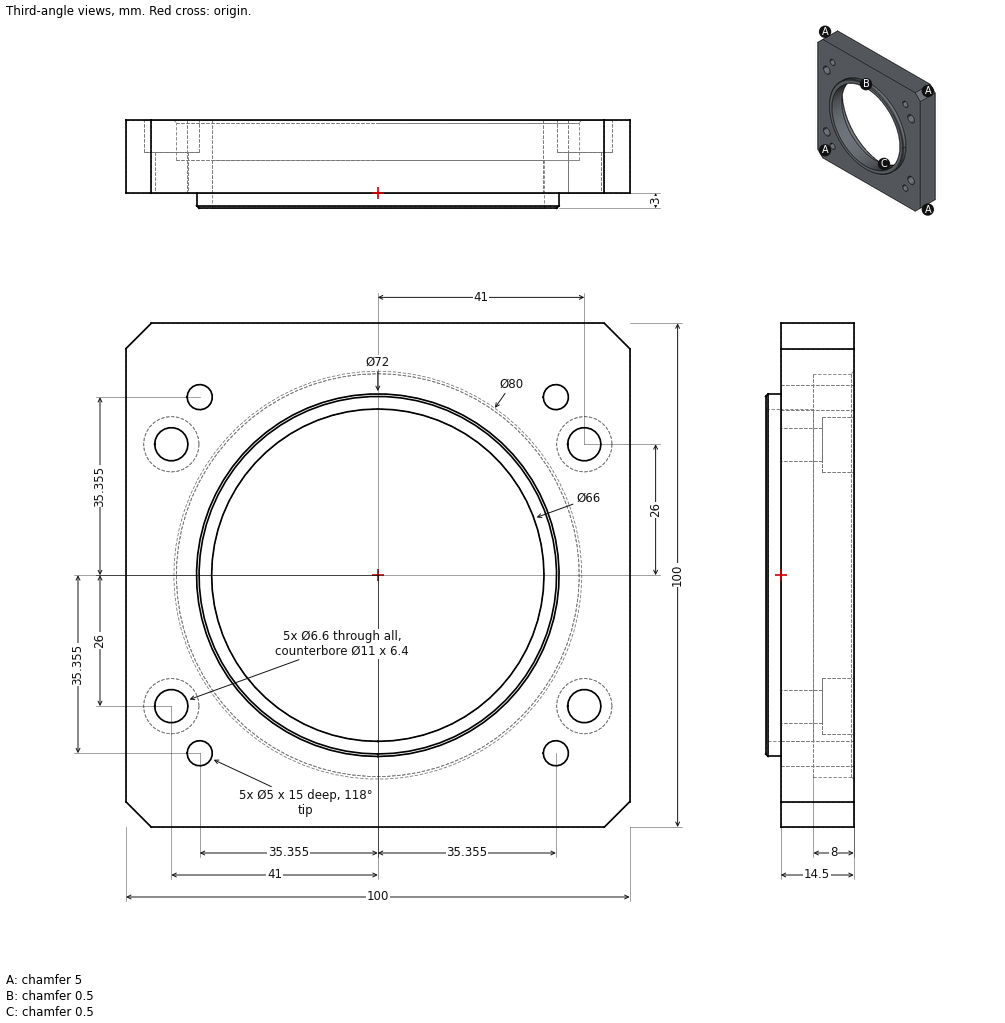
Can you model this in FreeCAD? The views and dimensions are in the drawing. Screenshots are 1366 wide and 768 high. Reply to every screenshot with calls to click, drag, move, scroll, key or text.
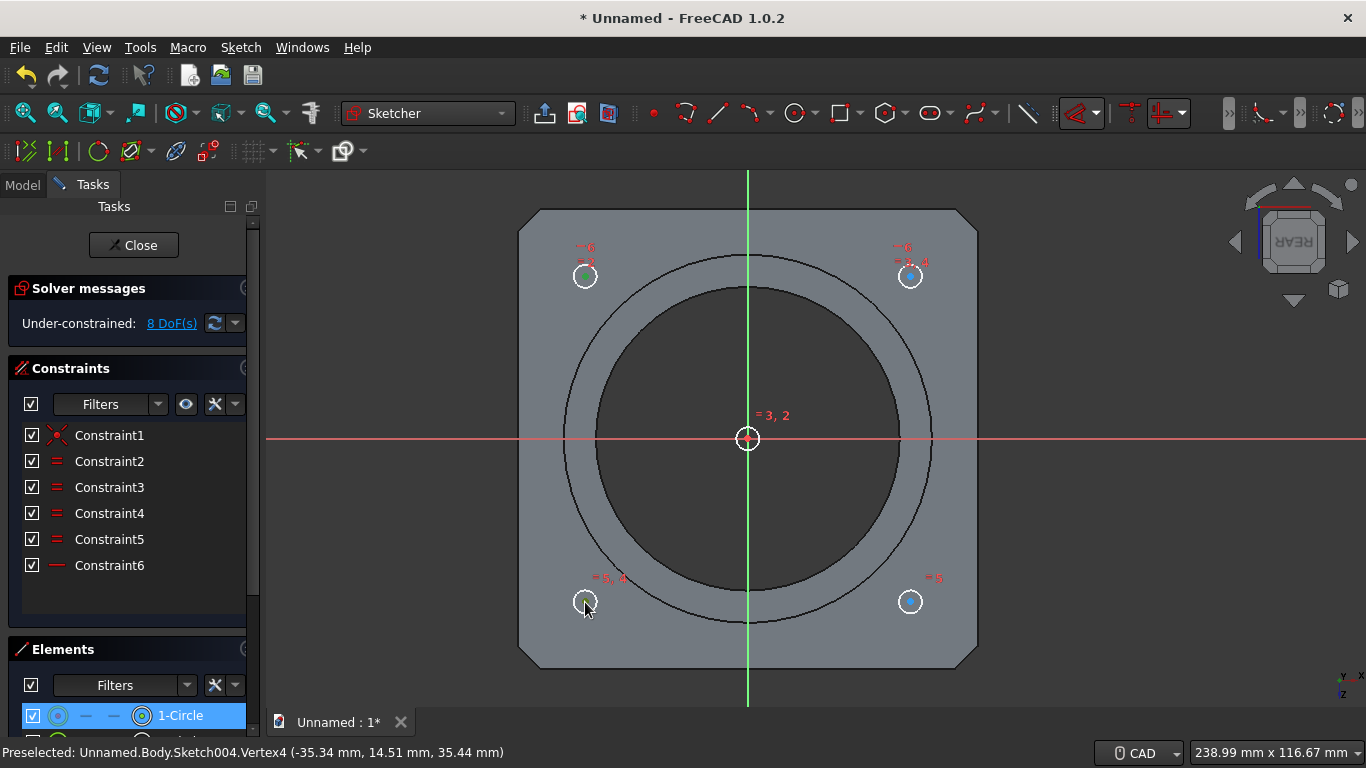
click(1184, 114)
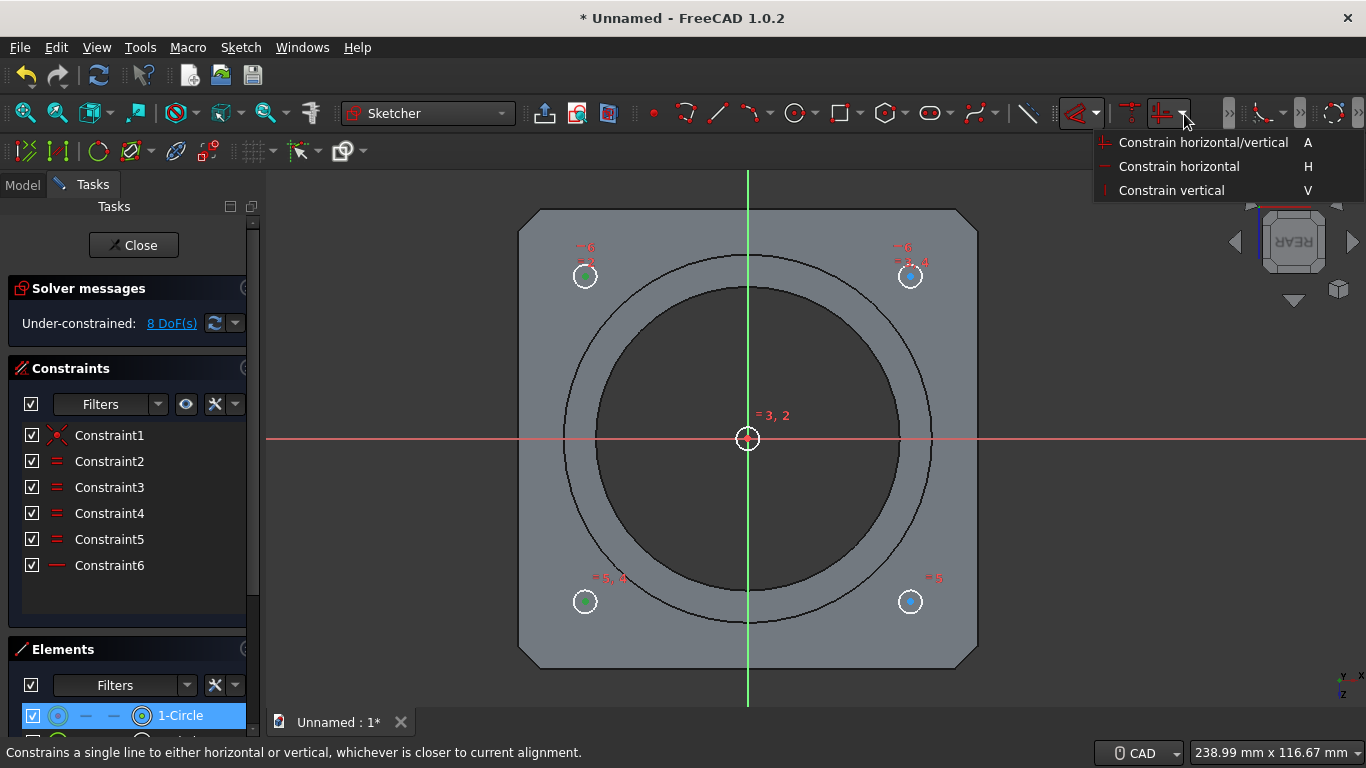
click(1229, 190)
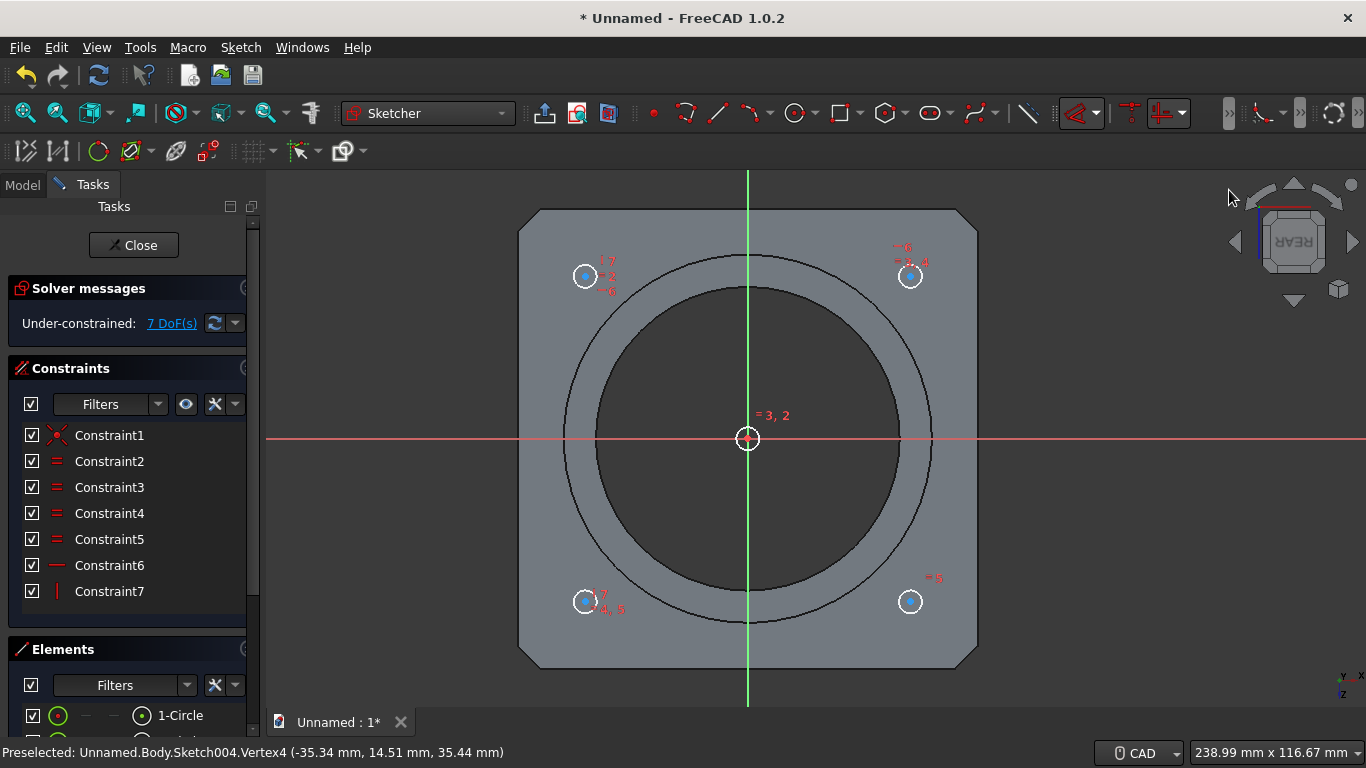
click(910, 276)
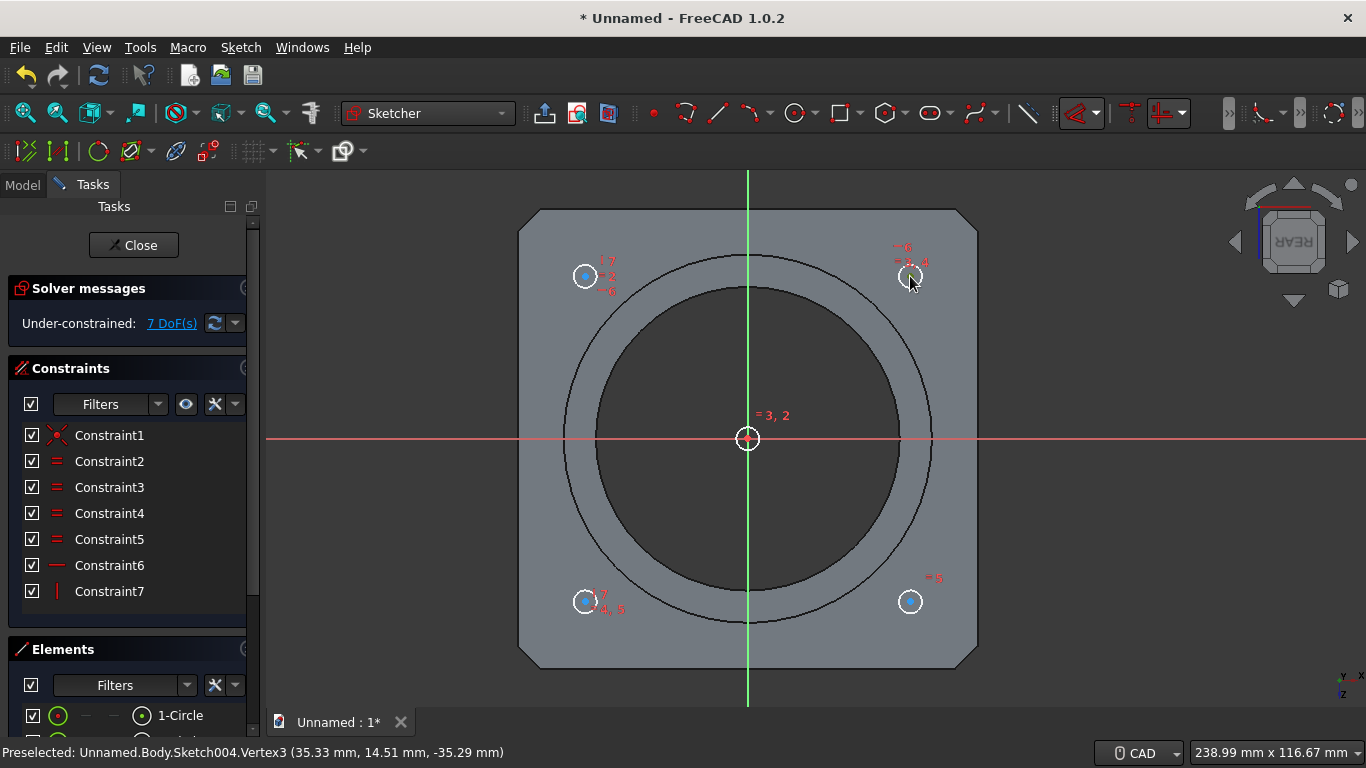
click(910, 602)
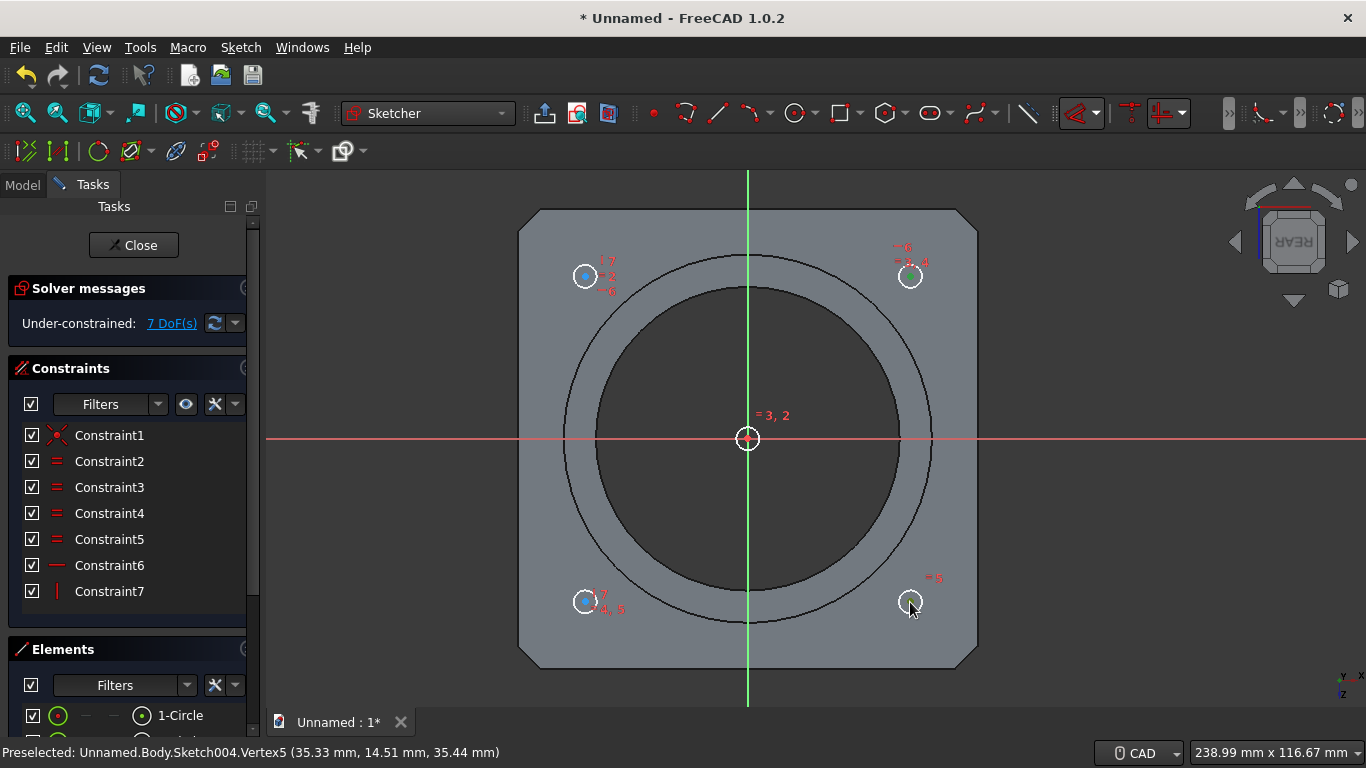
click(1184, 114)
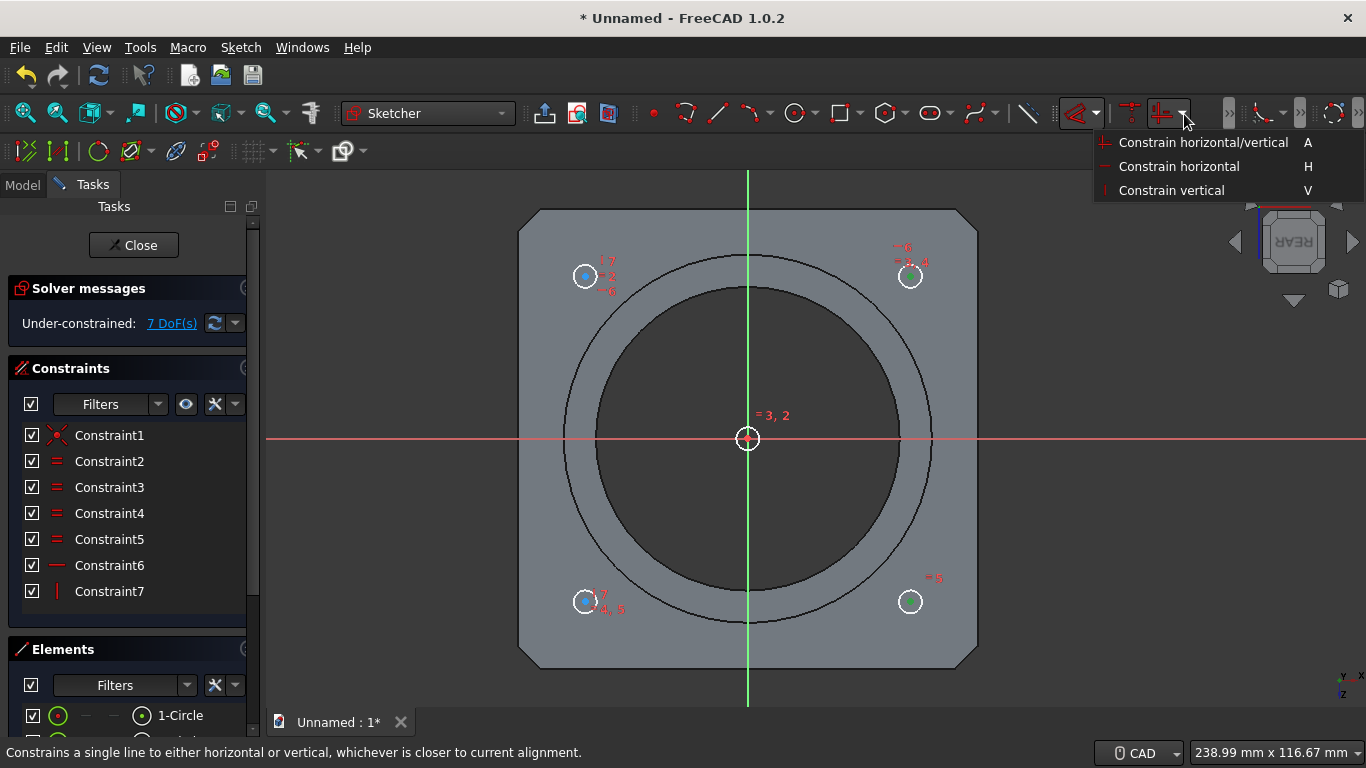
click(1229, 190)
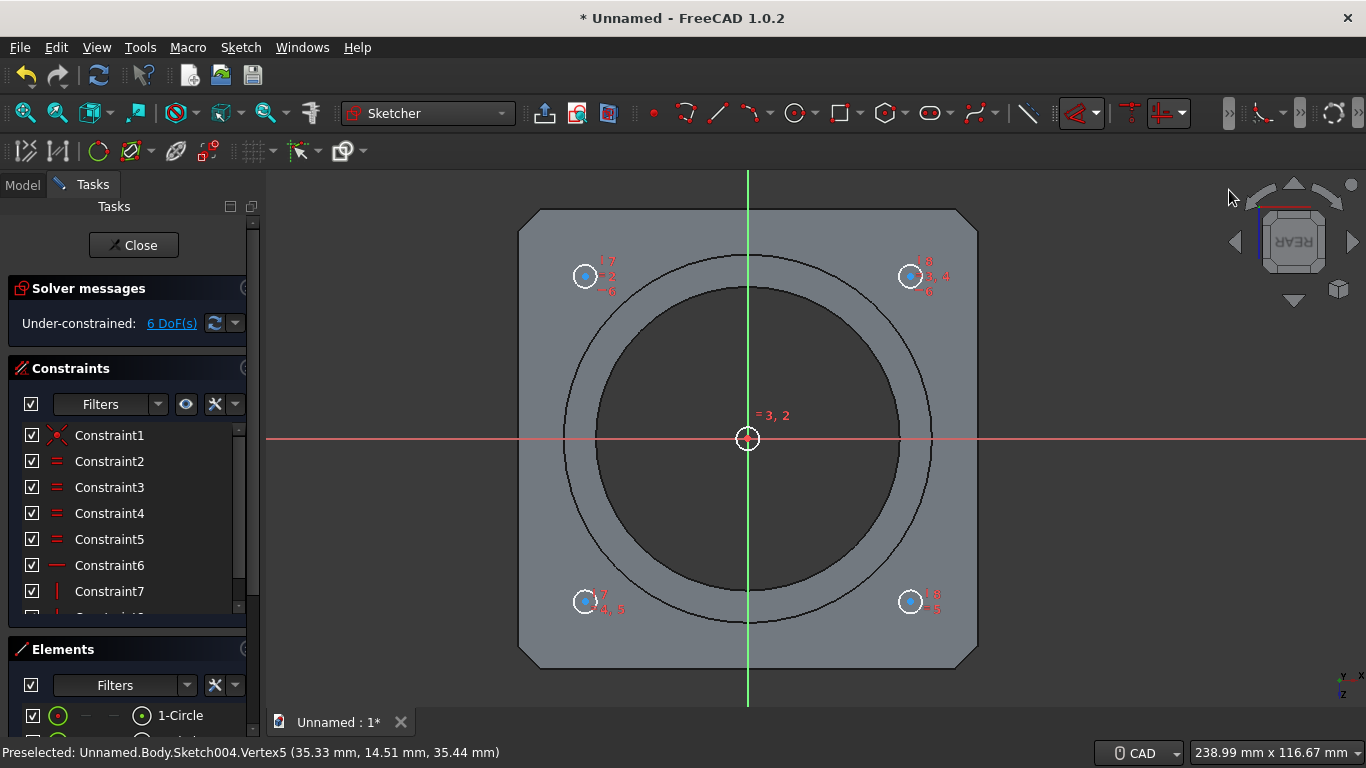
click(585, 602)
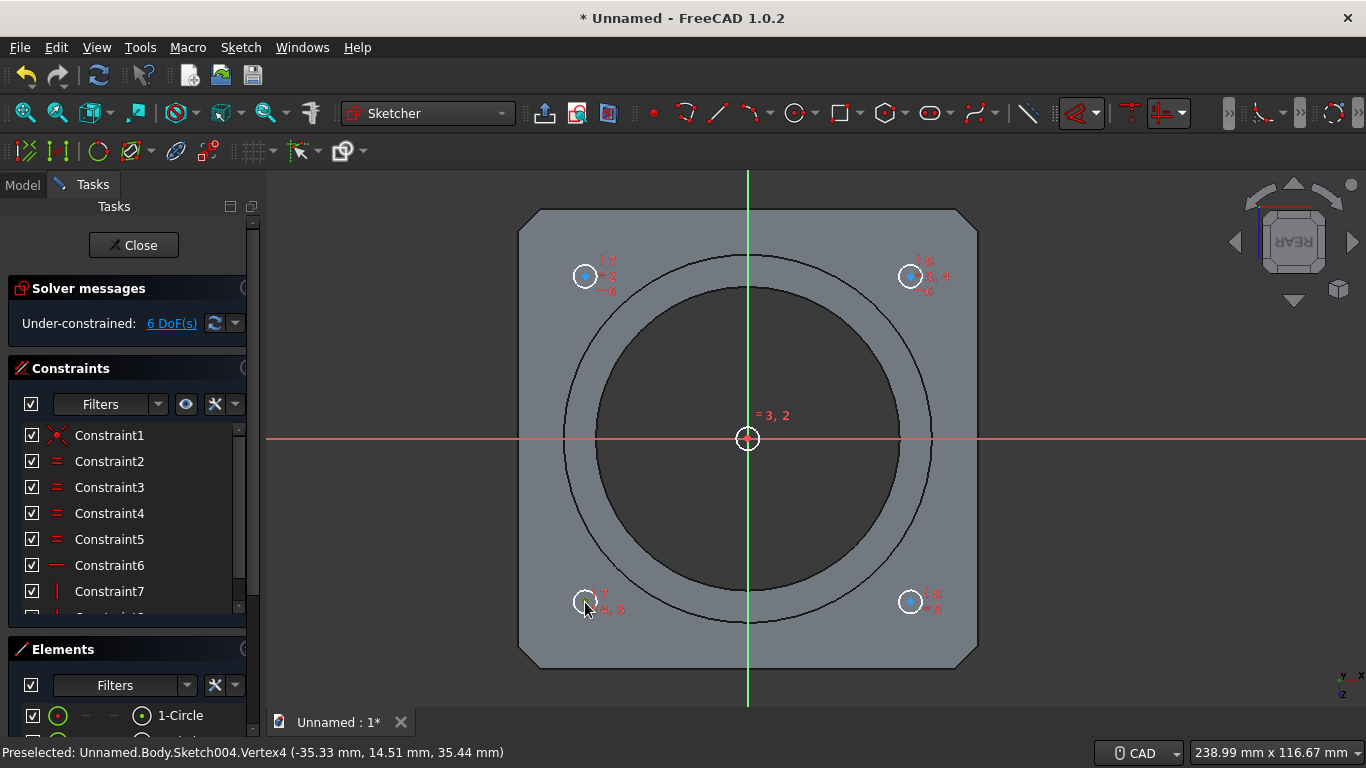
click(910, 602)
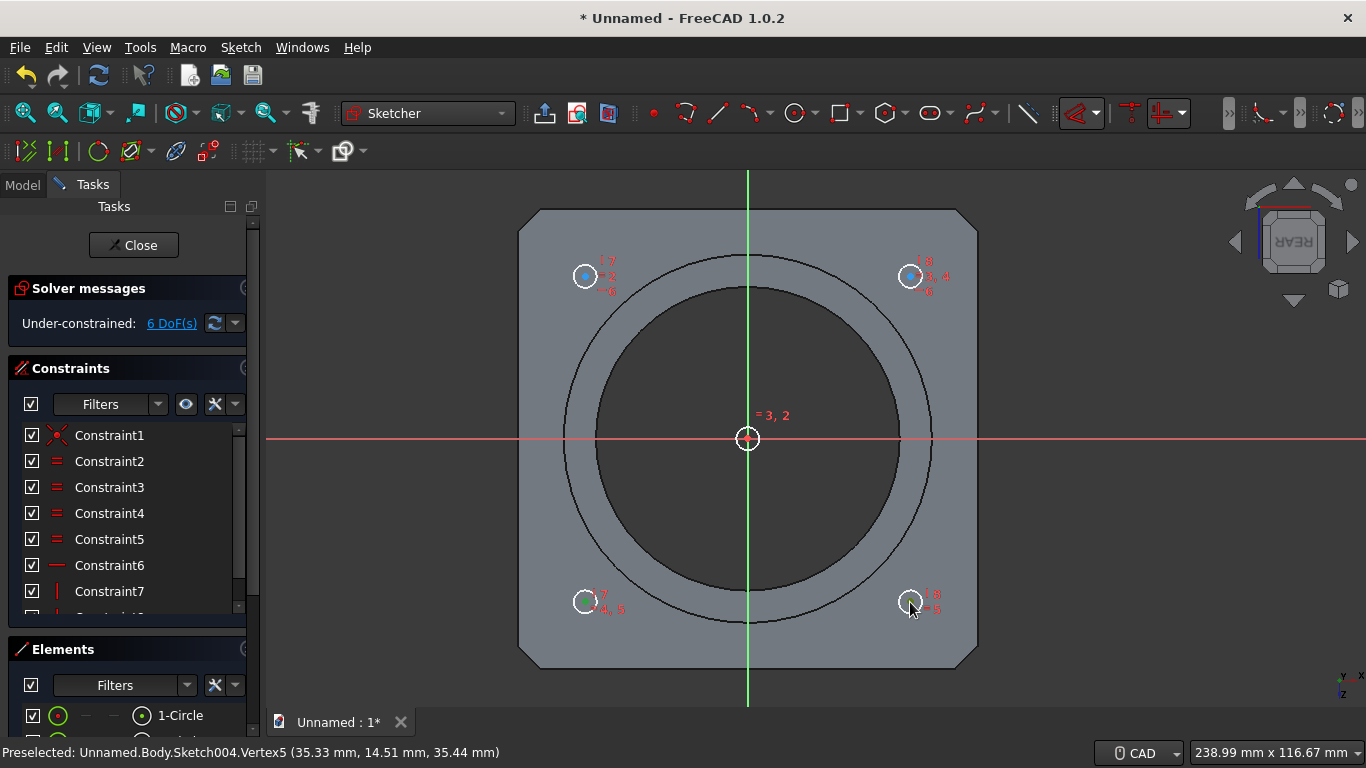
key(h)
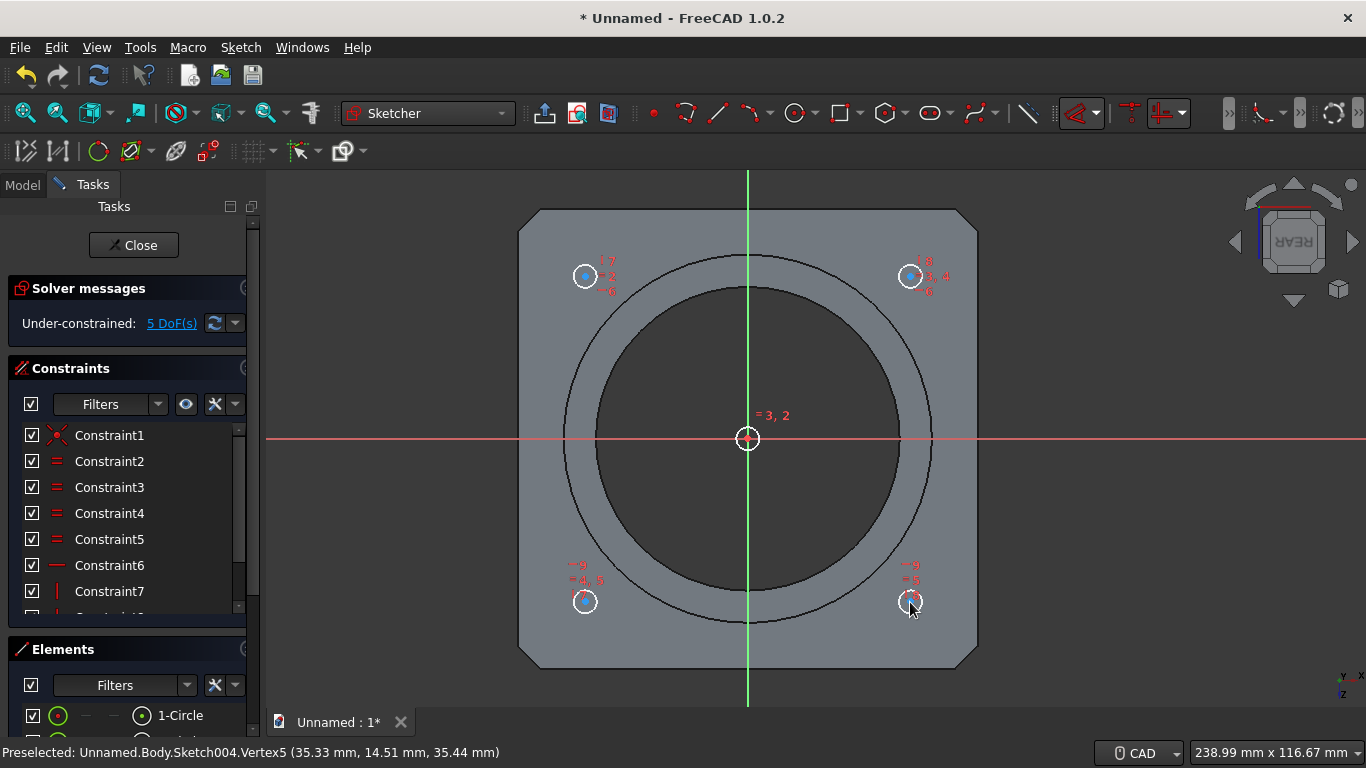
click(1076, 114)